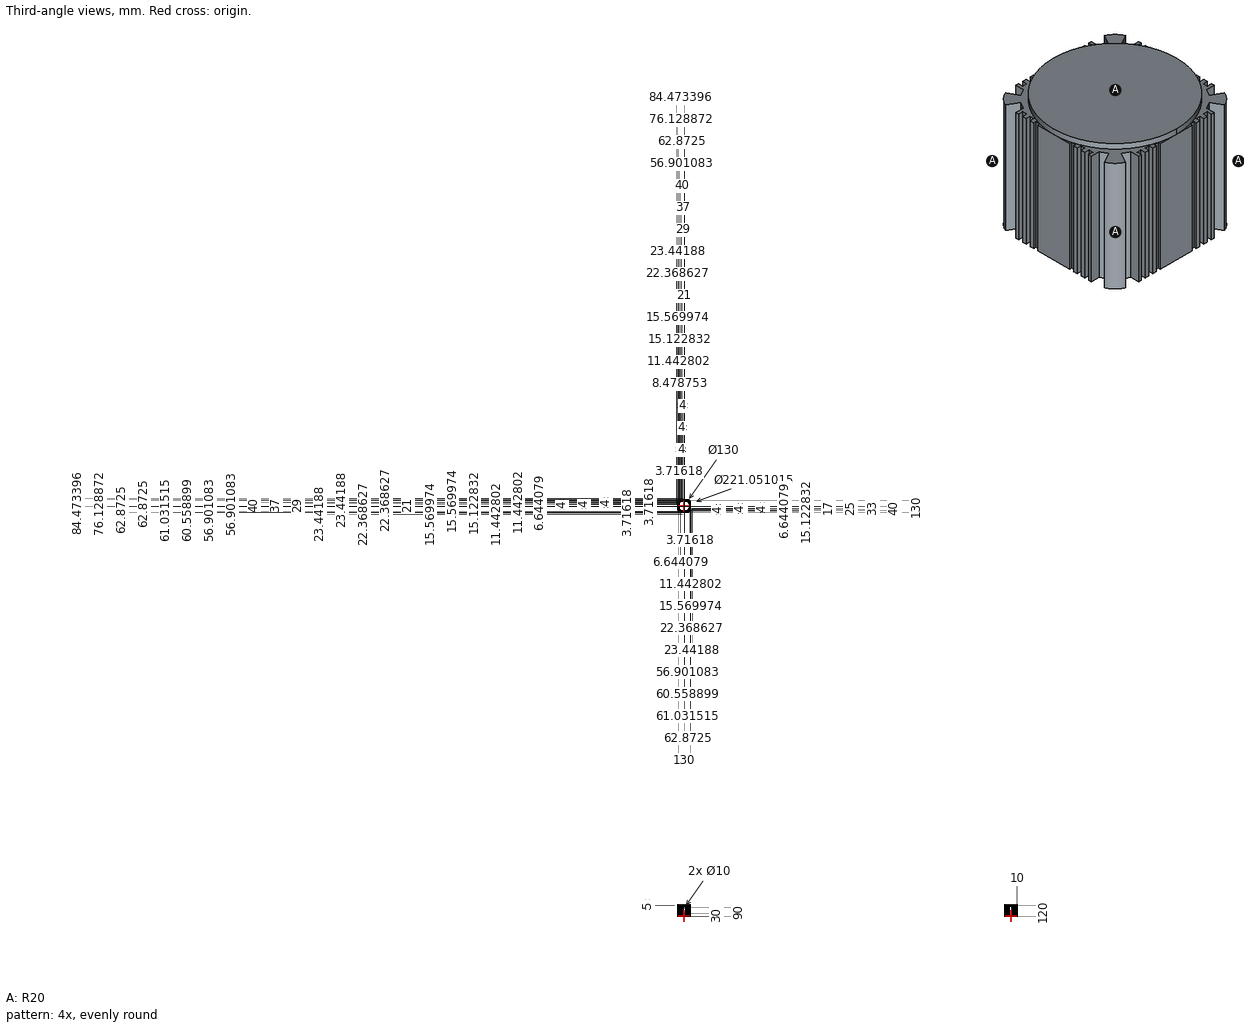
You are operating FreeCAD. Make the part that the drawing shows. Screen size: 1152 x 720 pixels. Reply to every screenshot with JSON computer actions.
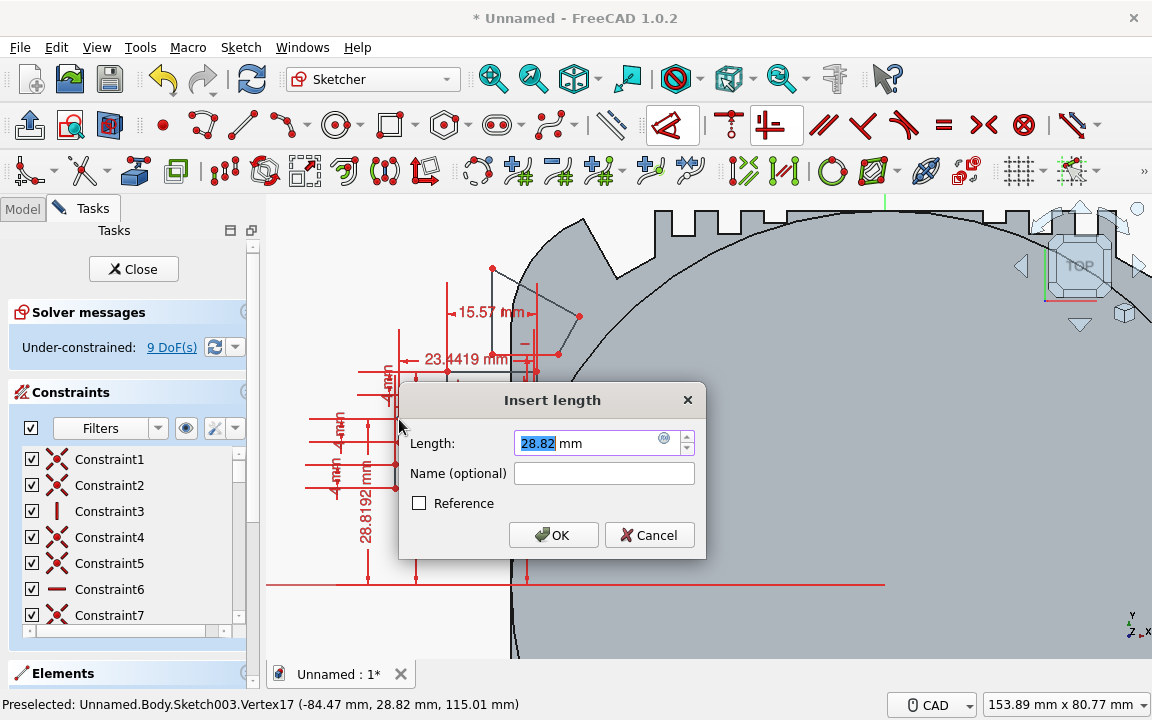
{"action": "type", "text": "29"}
{"action": "key", "text": "Return"}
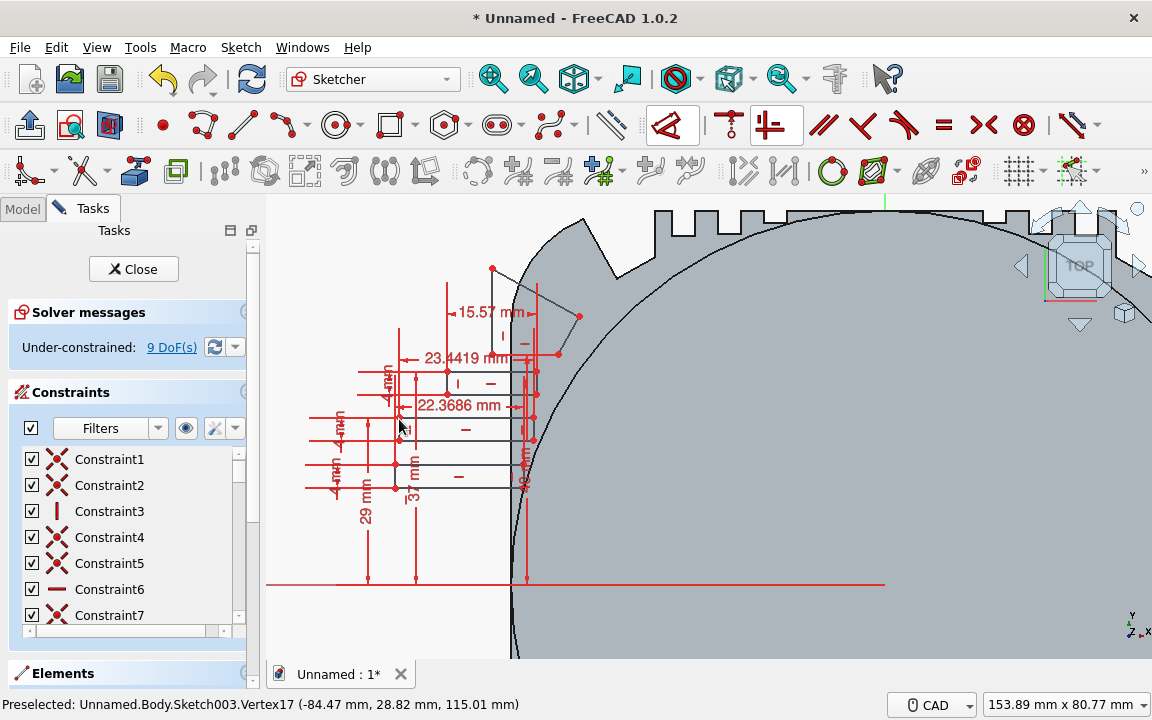
{"action": "left_click", "coordinate": [395, 465]}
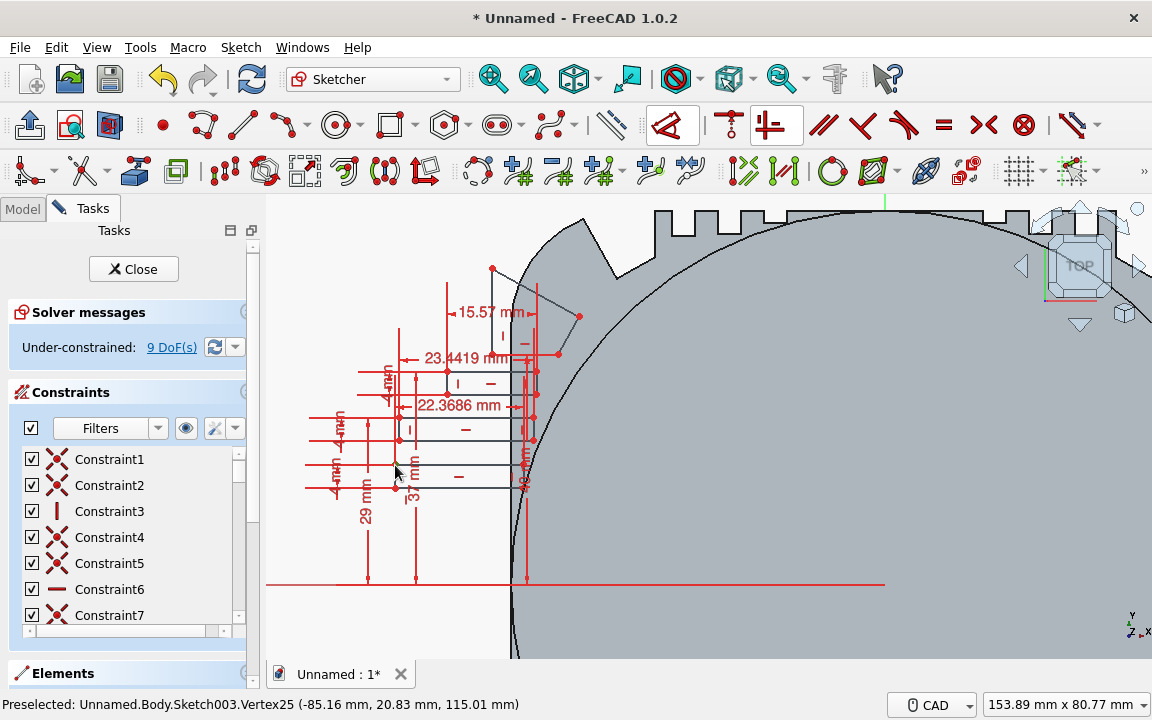
{"action": "left_click", "coordinate": [694, 126]}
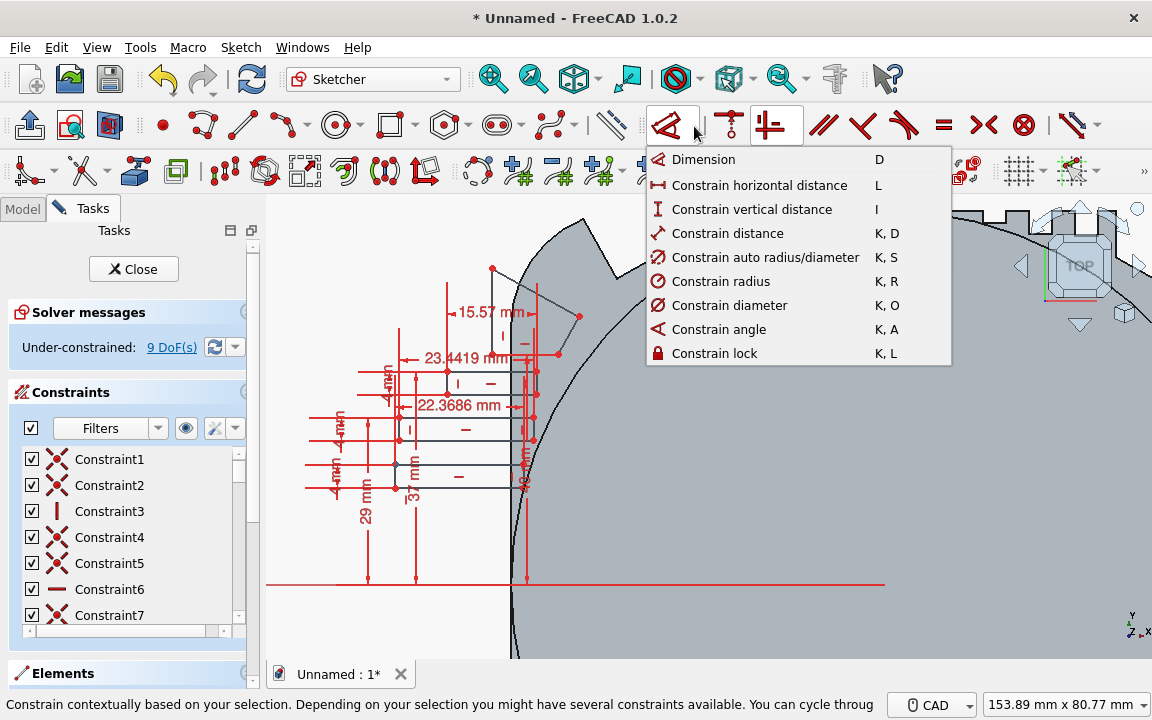
{"action": "left_click", "coordinate": [799, 209]}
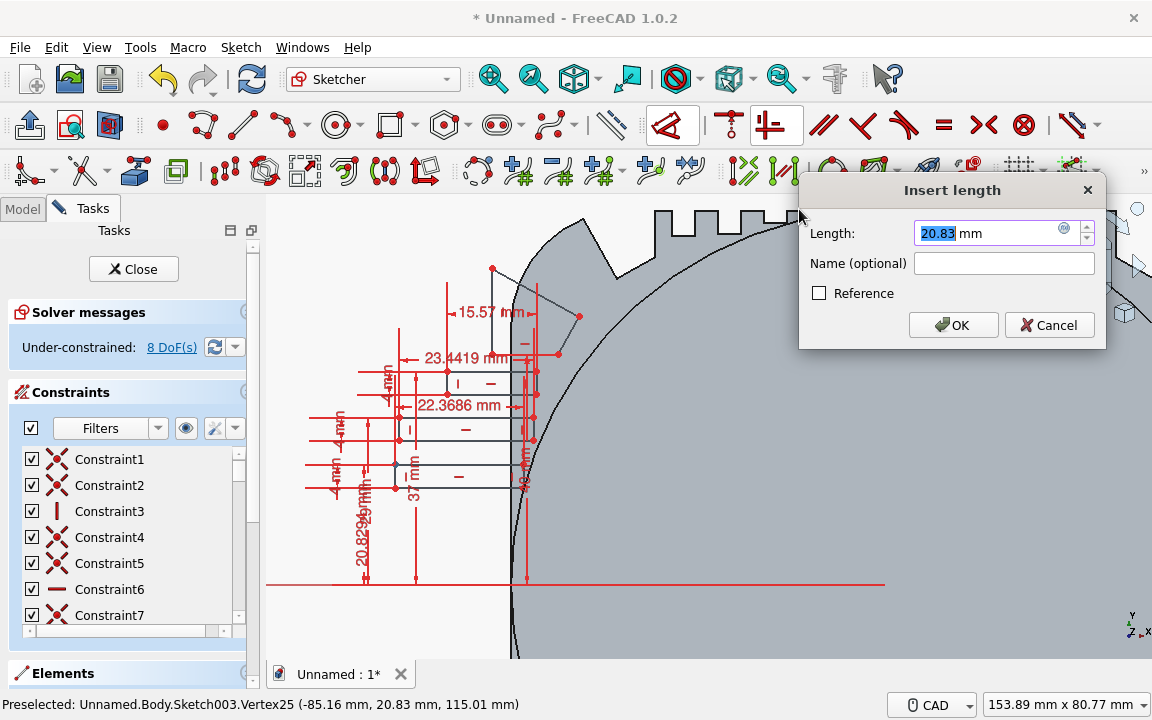
{"action": "type", "text": "21"}
{"action": "key", "text": "Return"}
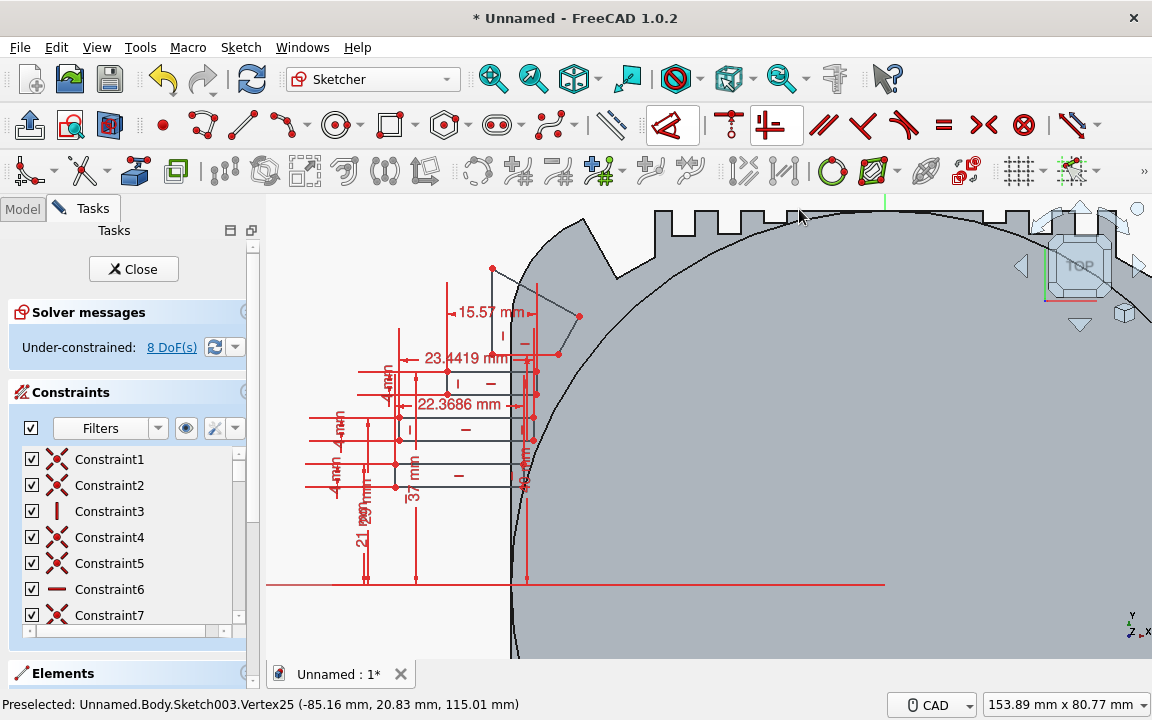
{"action": "left_click", "coordinate": [524, 487]}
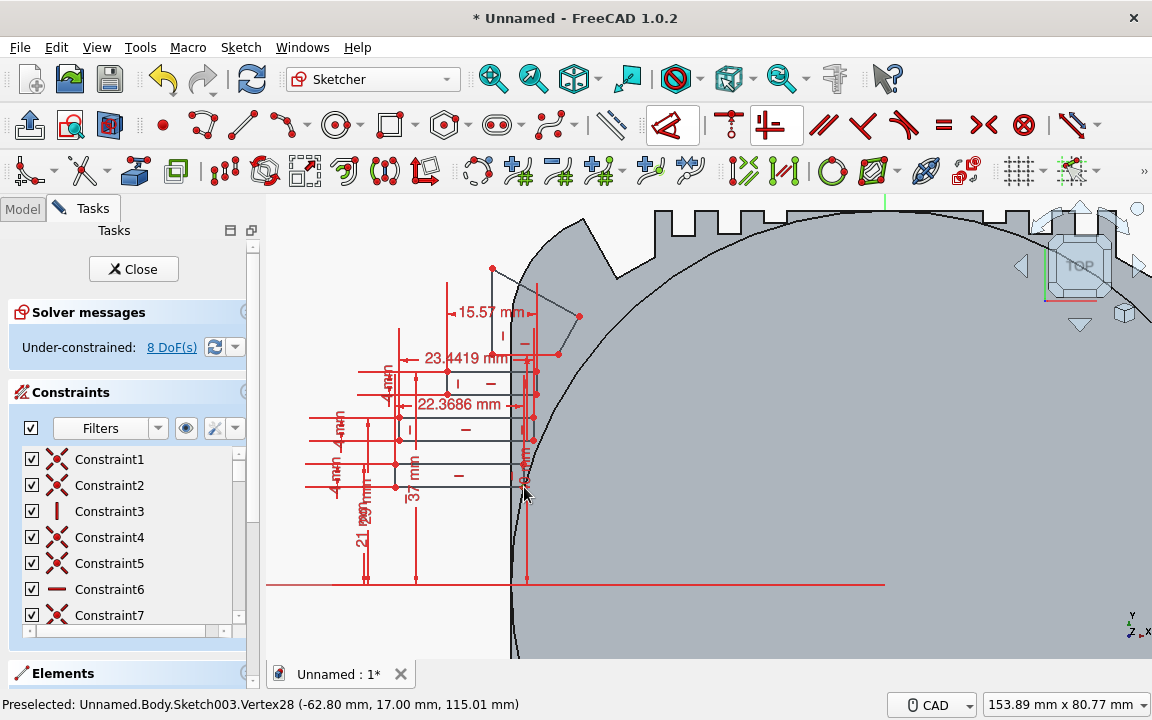
{"action": "key", "text": "l"}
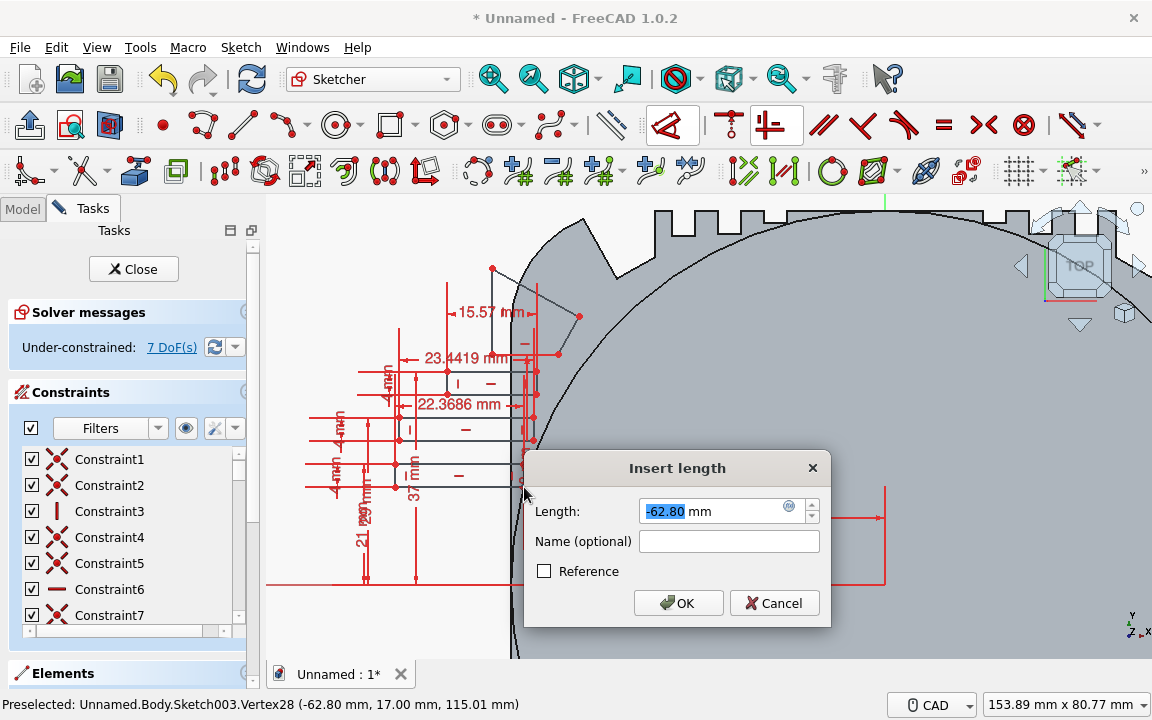
{"action": "type", "text": "-62.8725"}
{"action": "key", "text": "Return"}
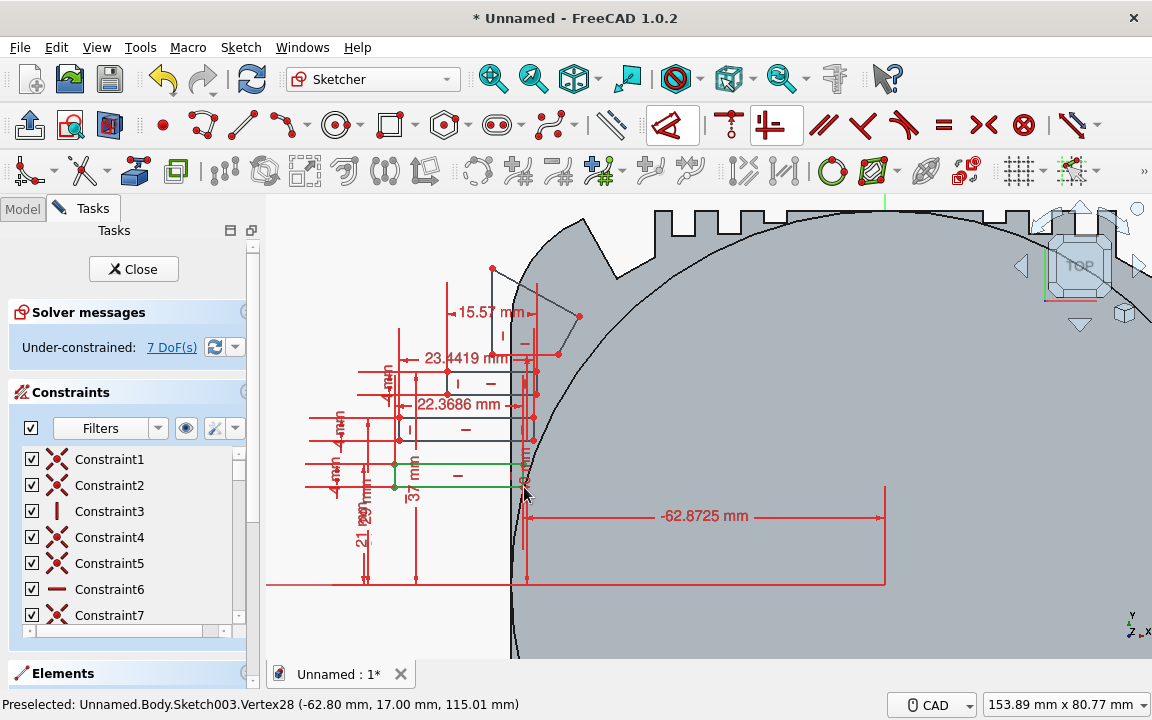
{"action": "scroll", "coordinate": [564, 343], "scroll_direction": "up", "scroll_amount": 4}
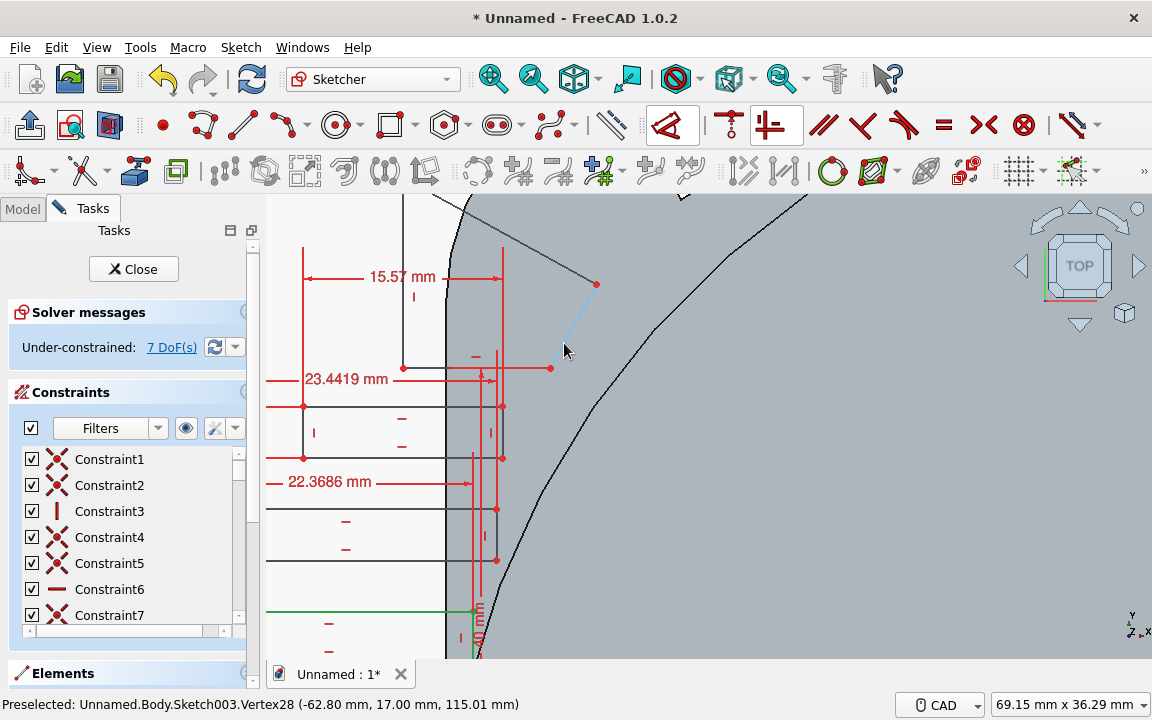
{"action": "left_click", "coordinate": [564, 343]}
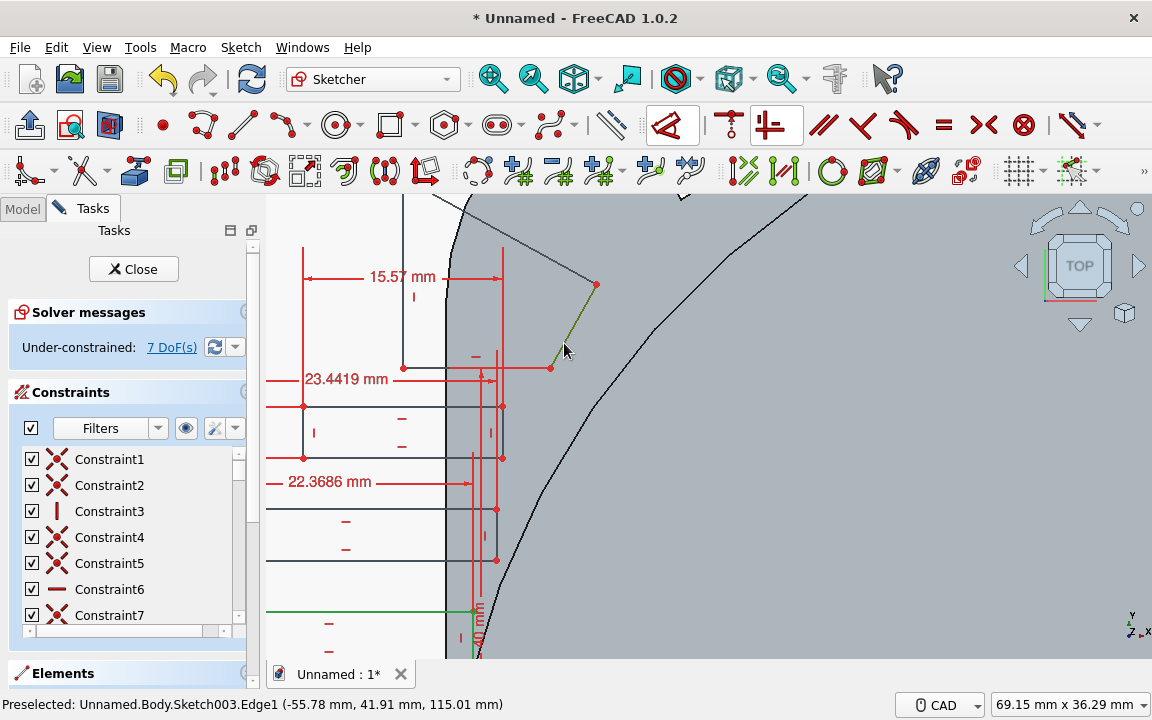
{"action": "left_click", "coordinate": [694, 126]}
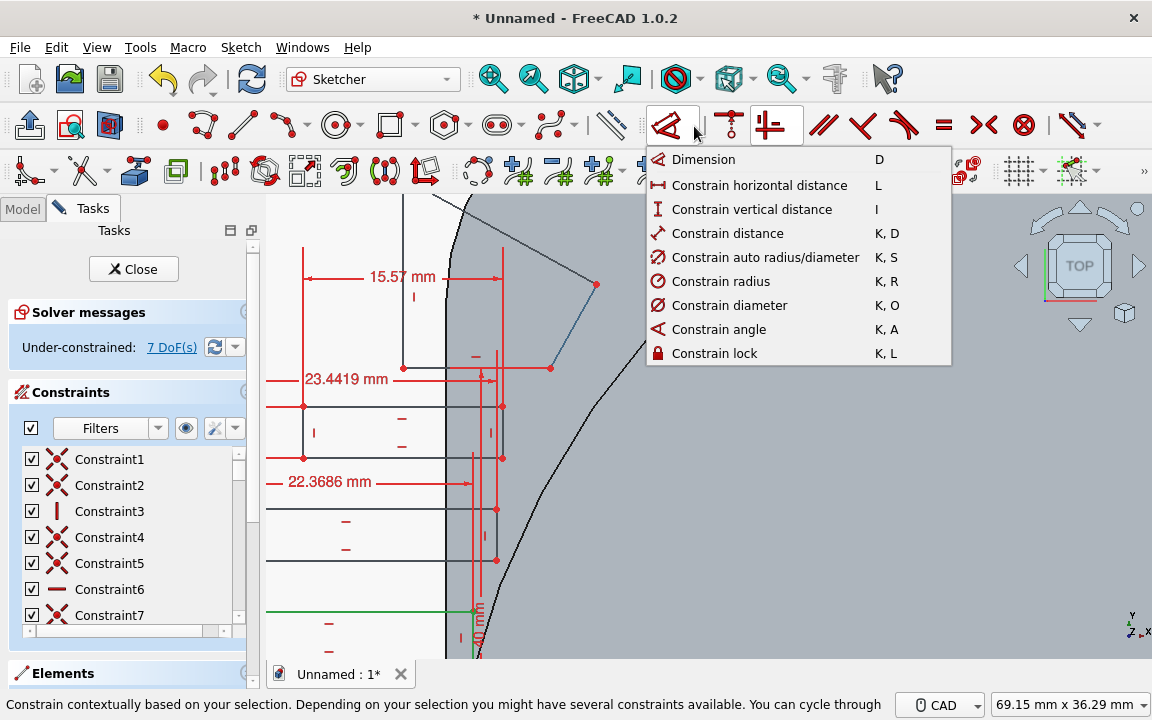
{"action": "left_click", "coordinate": [799, 185]}